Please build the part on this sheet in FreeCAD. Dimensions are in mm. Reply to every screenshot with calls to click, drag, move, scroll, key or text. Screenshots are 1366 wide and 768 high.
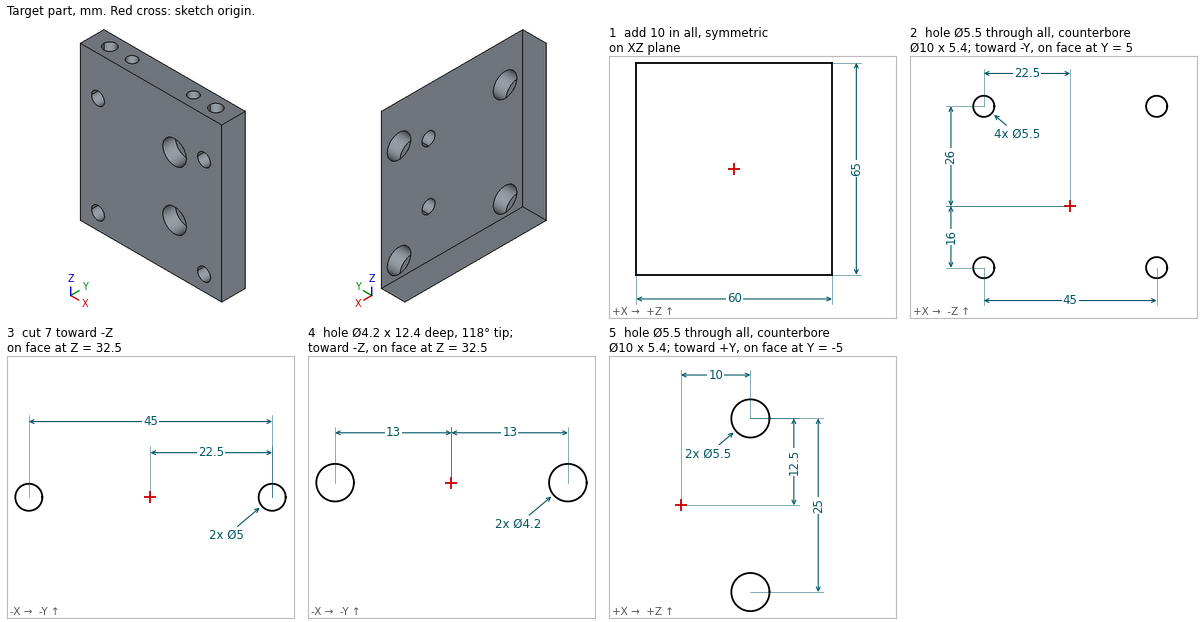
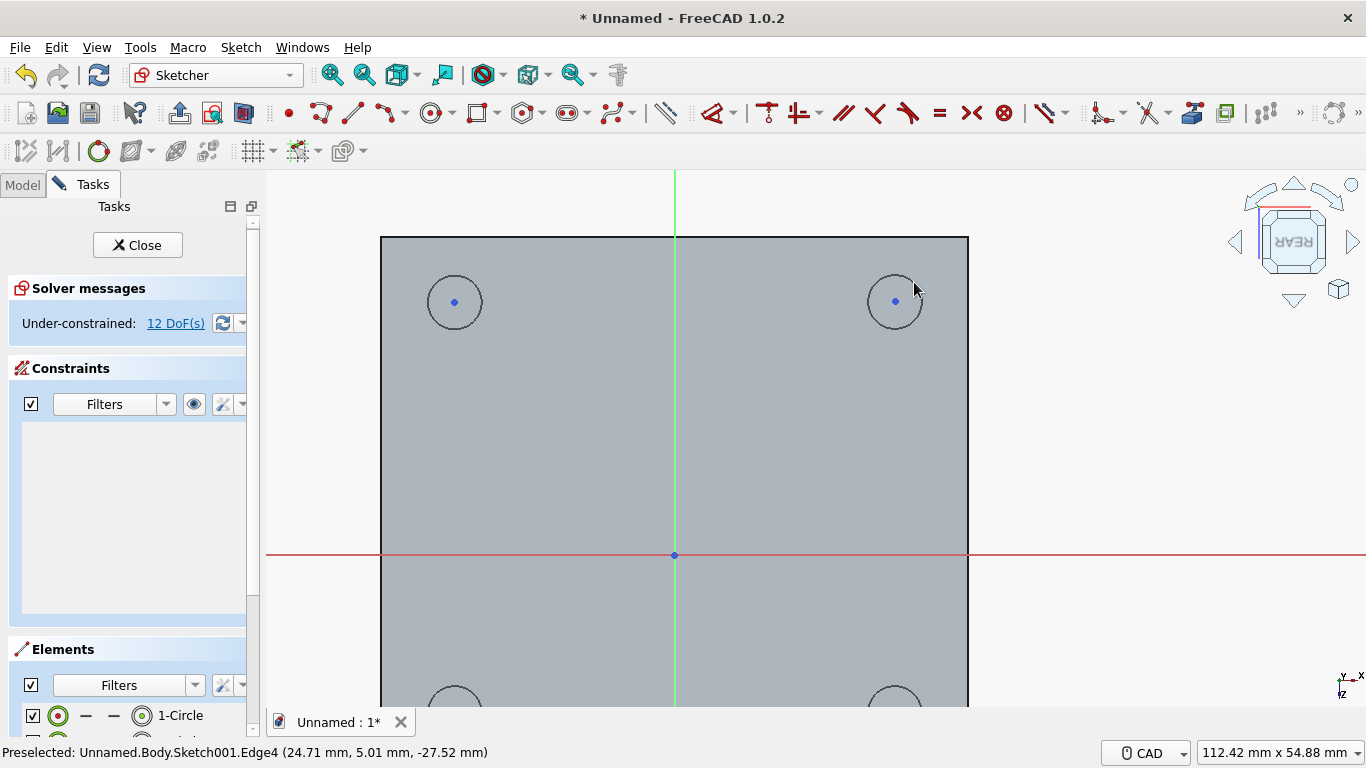
click(474, 283)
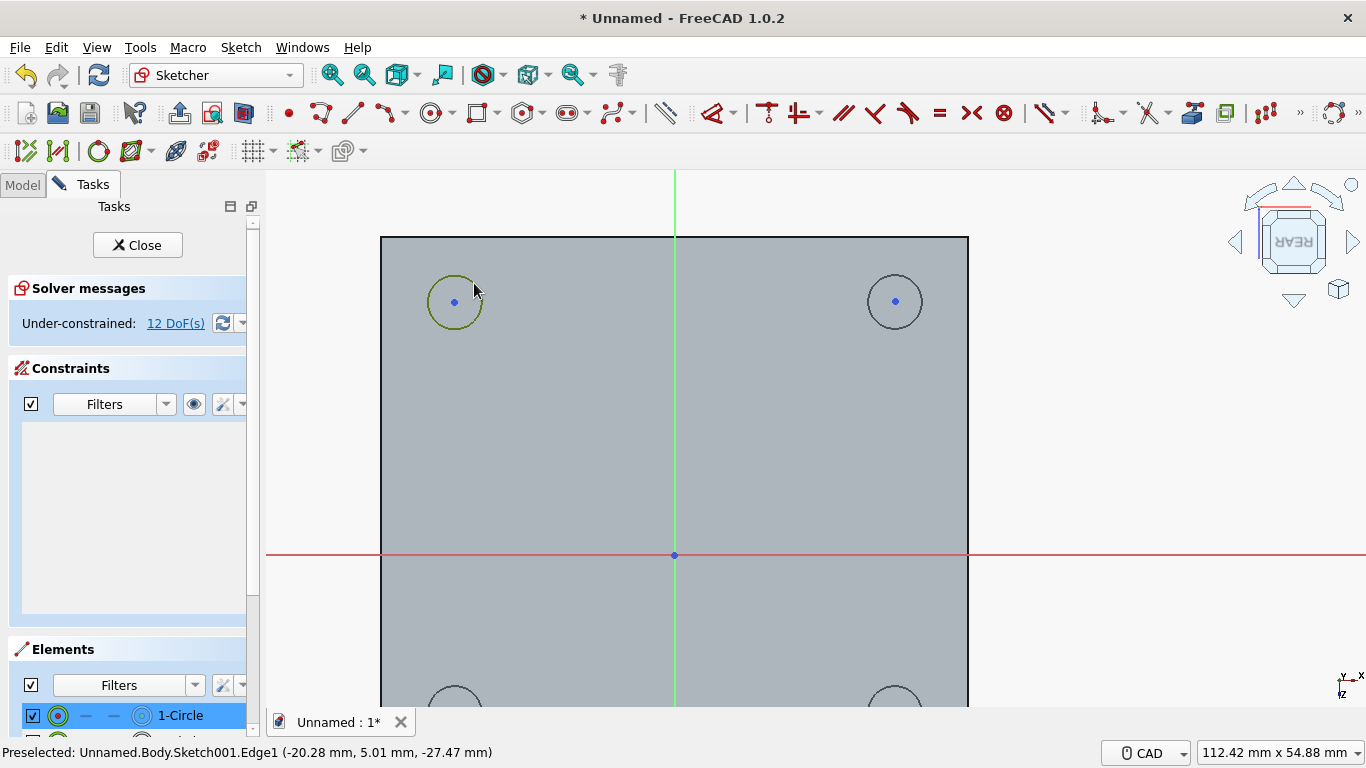
scroll(895, 300, down, 2)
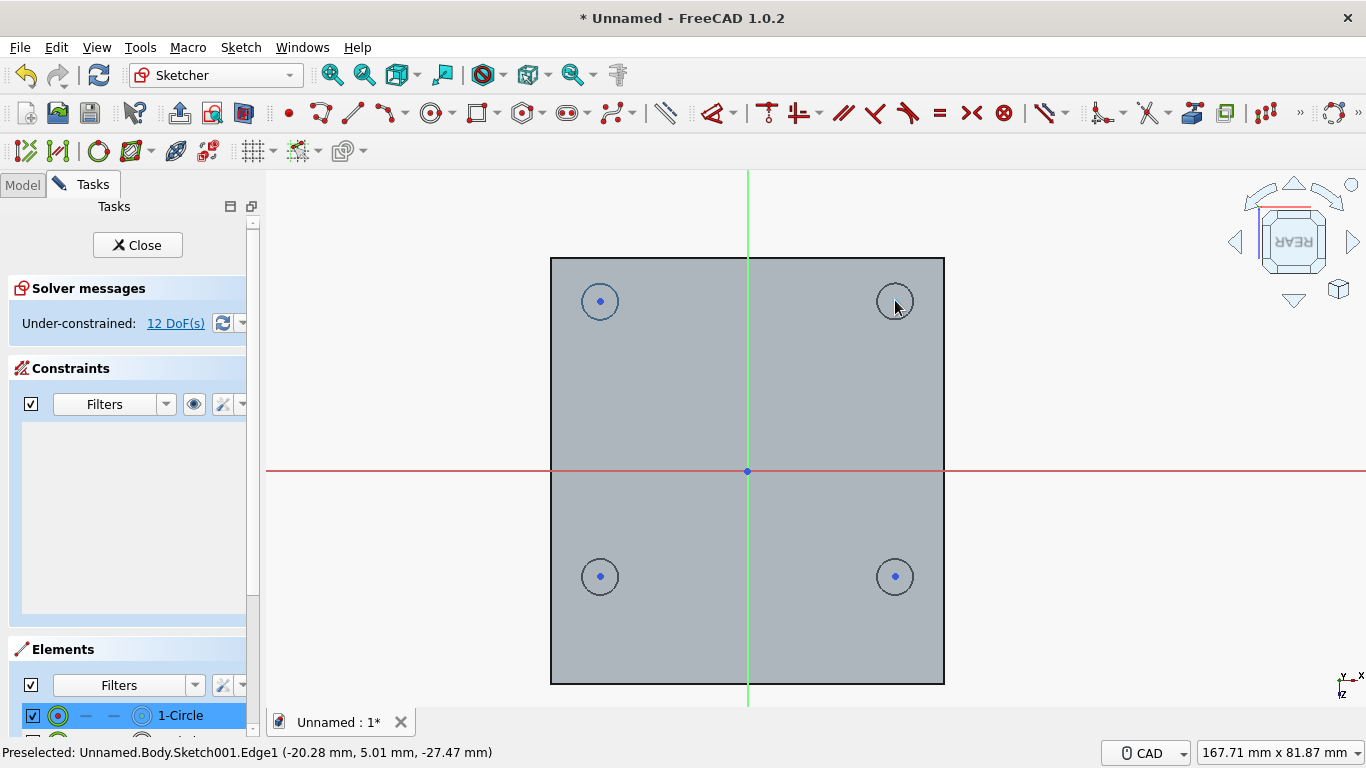
click(613, 564)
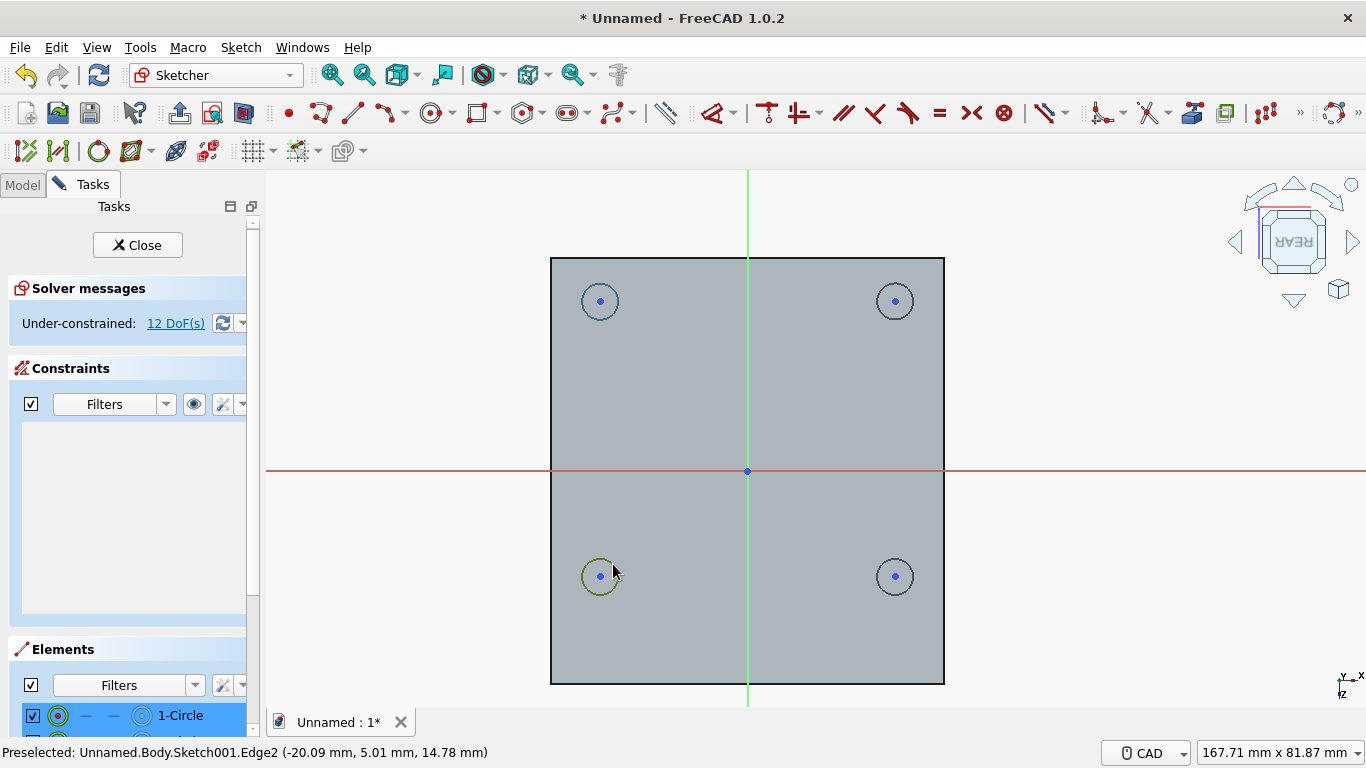
click(908, 564)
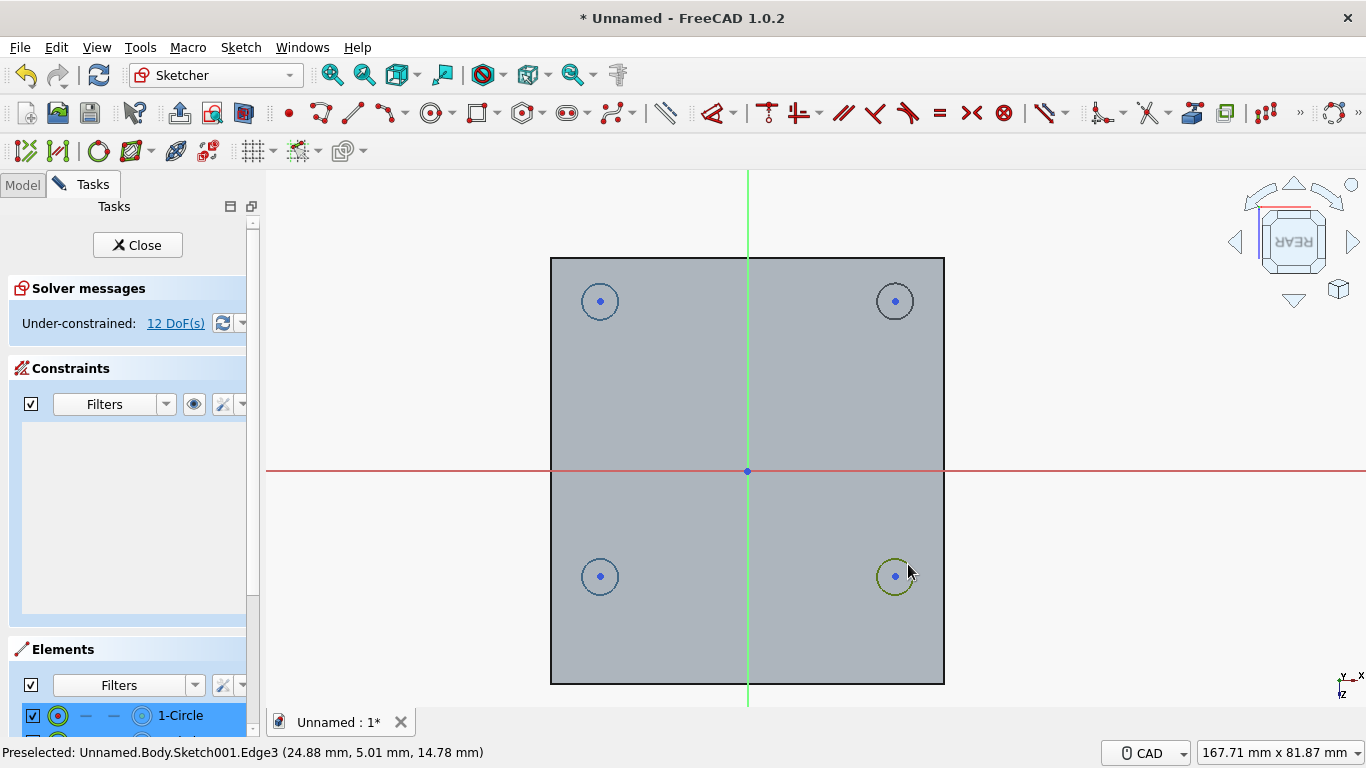
click(908, 289)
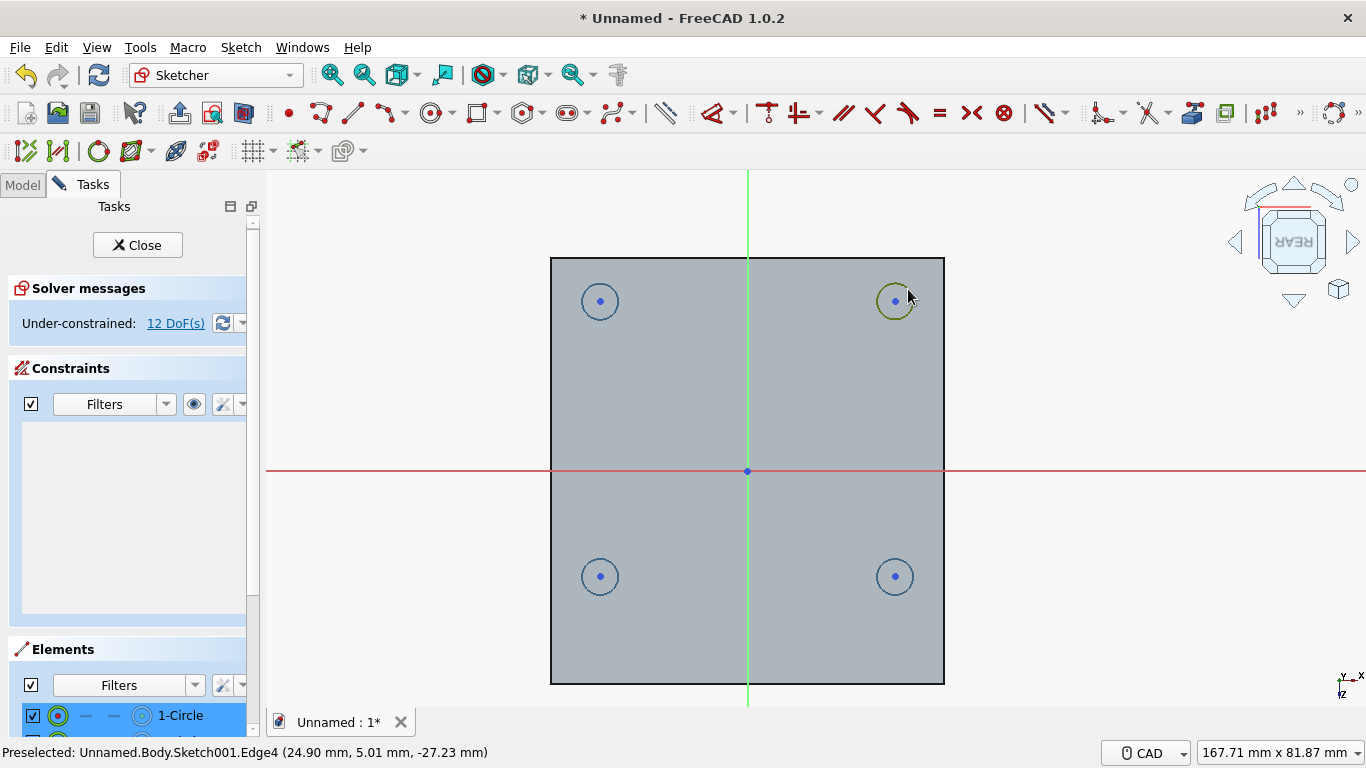
key(e)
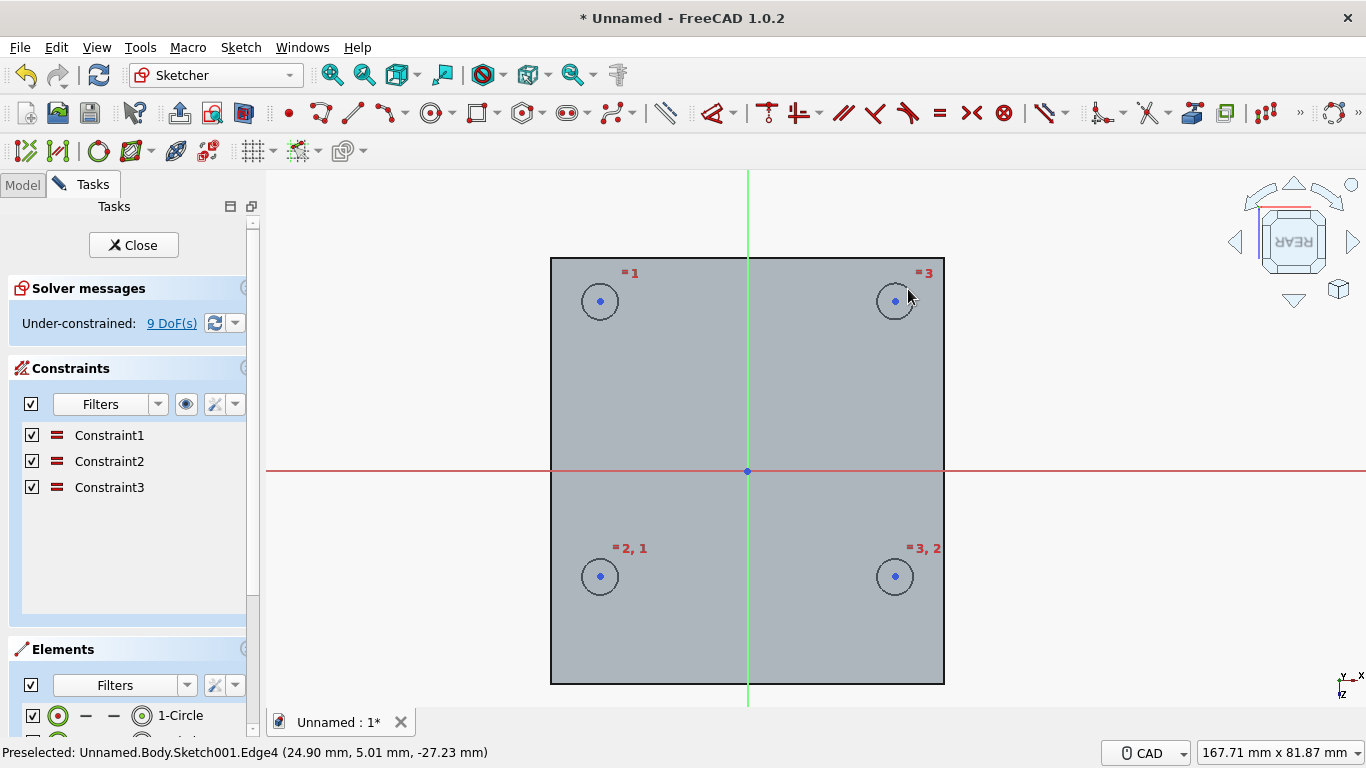
click(600, 302)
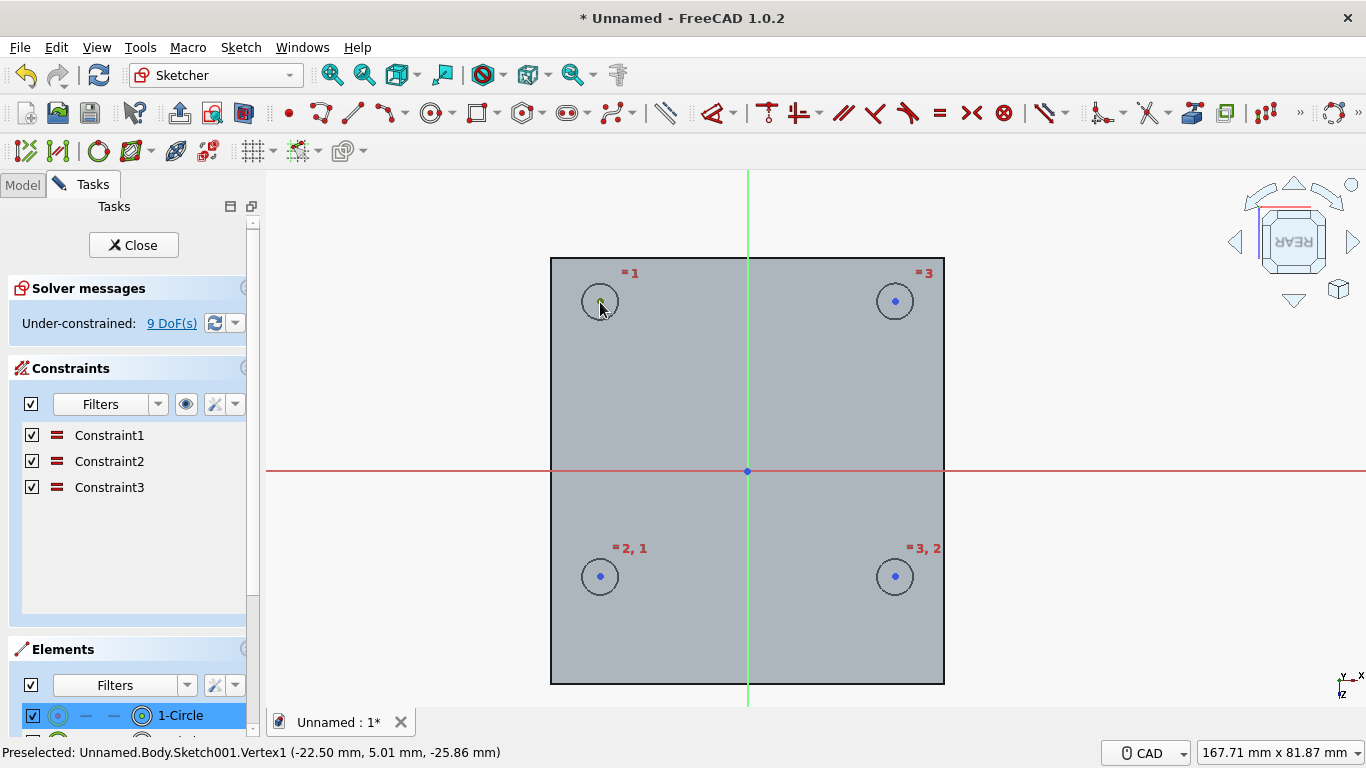
click(600, 577)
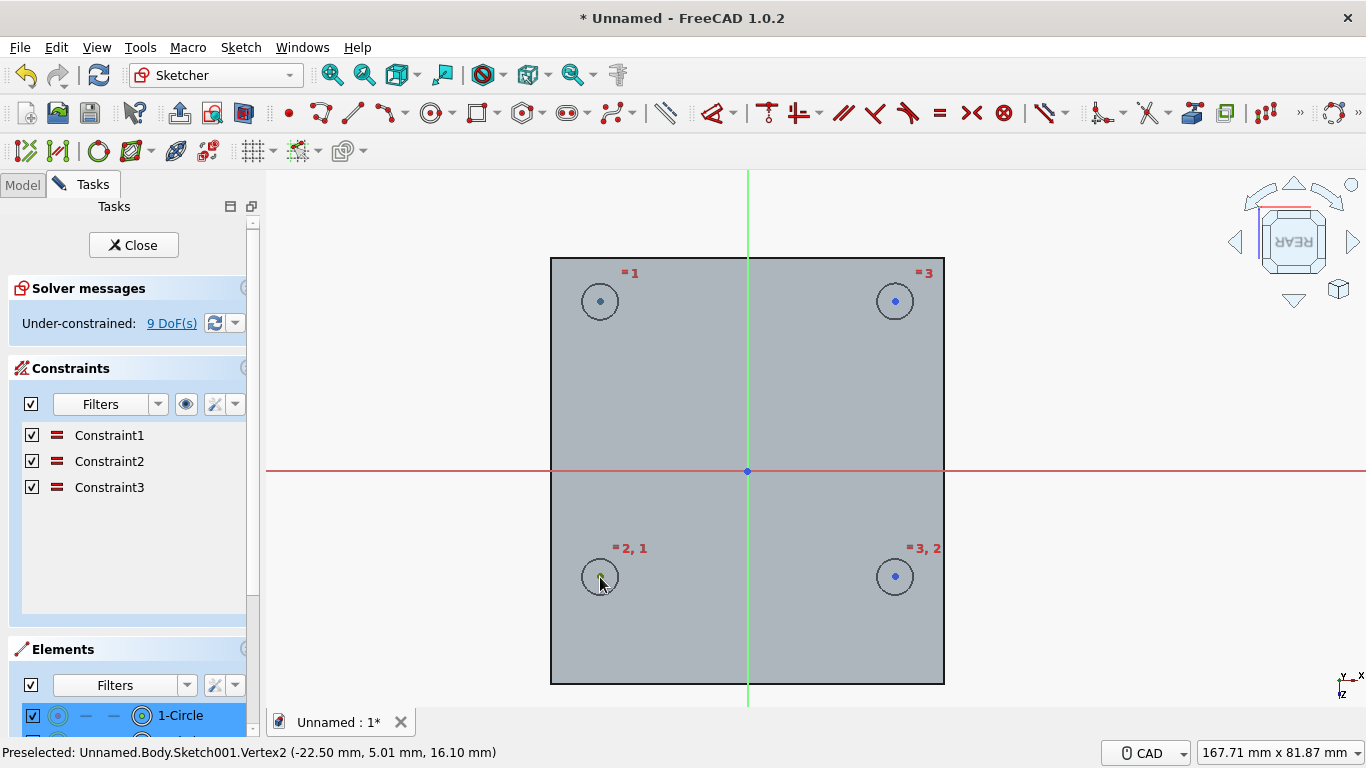
key(v)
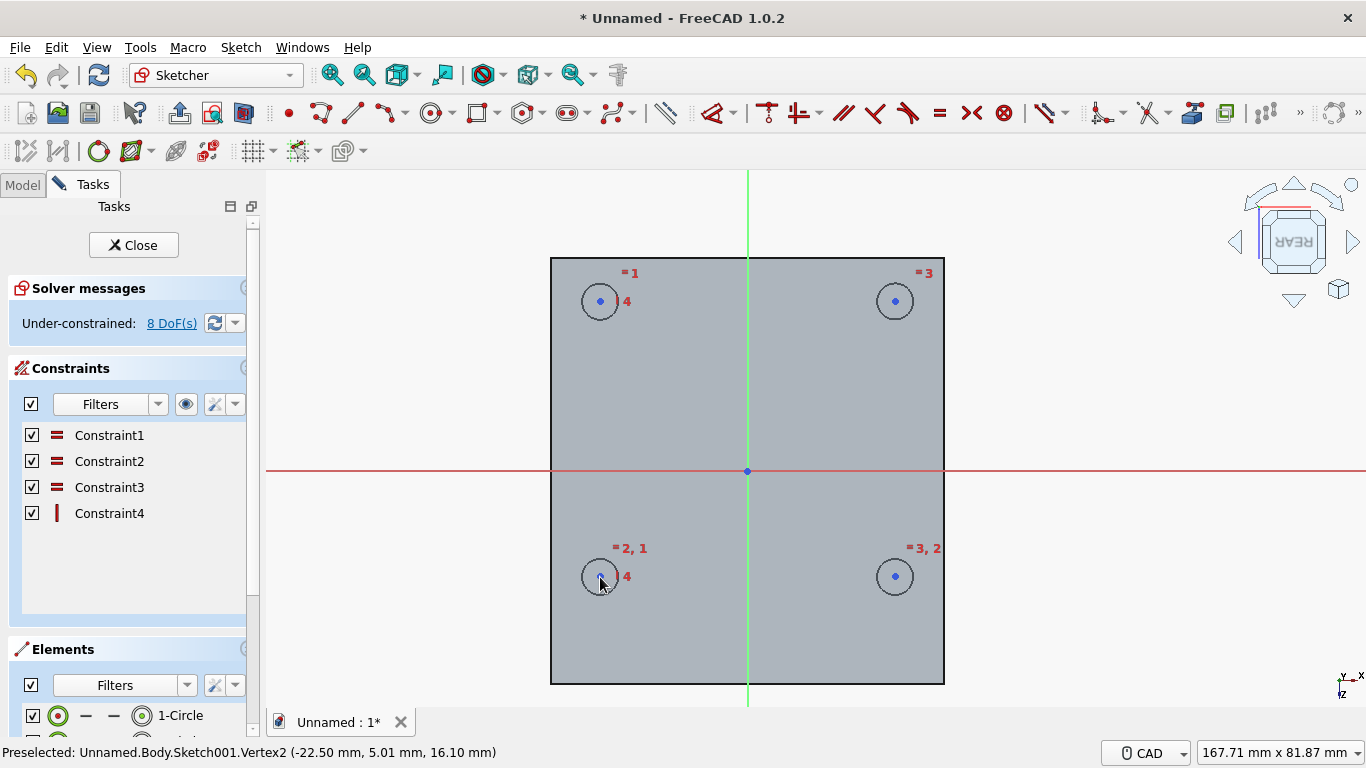
click(600, 577)